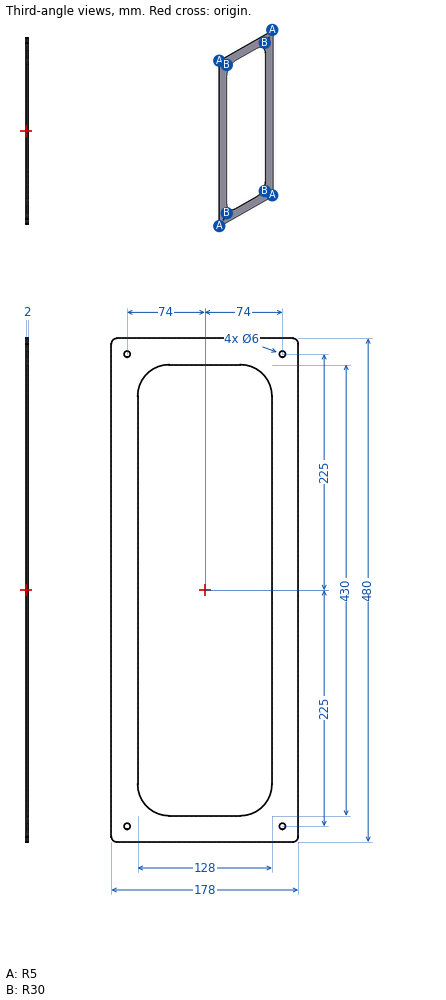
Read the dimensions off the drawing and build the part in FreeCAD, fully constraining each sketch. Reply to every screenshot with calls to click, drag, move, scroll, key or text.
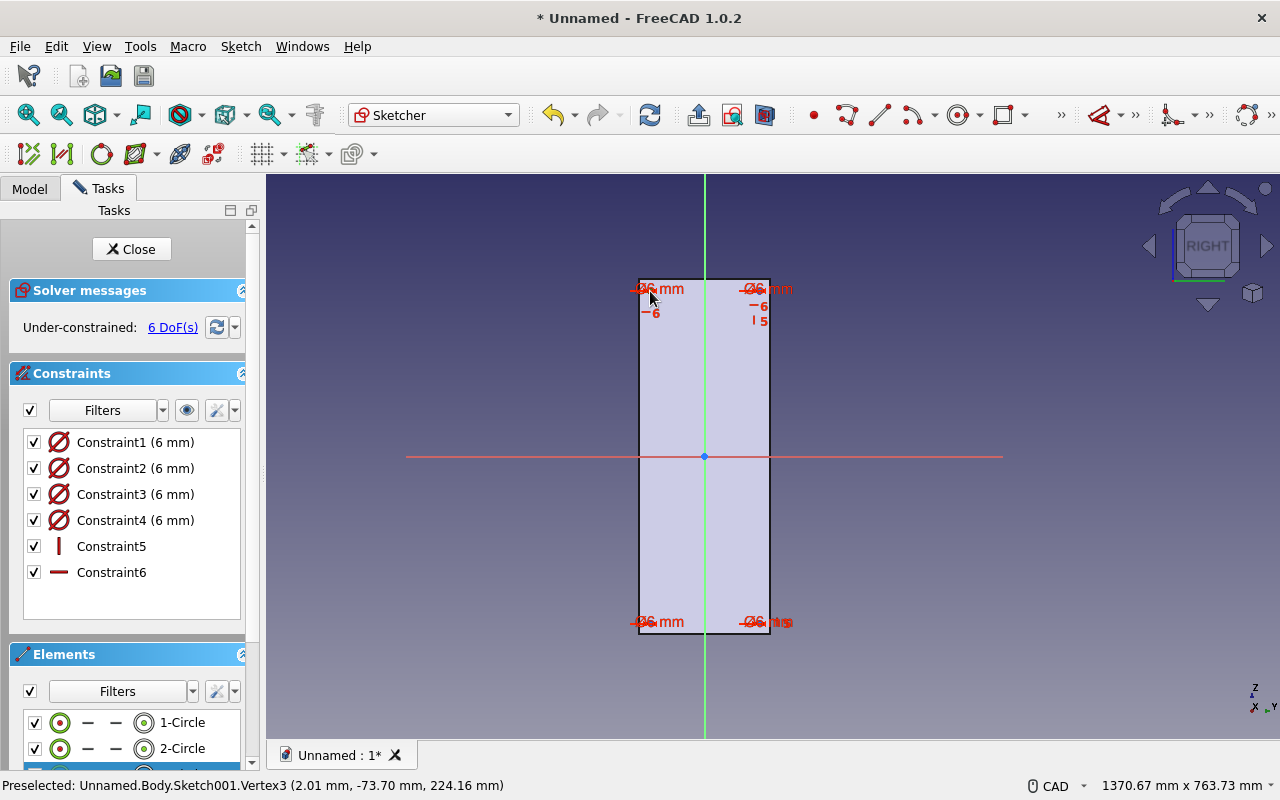
click(650, 624)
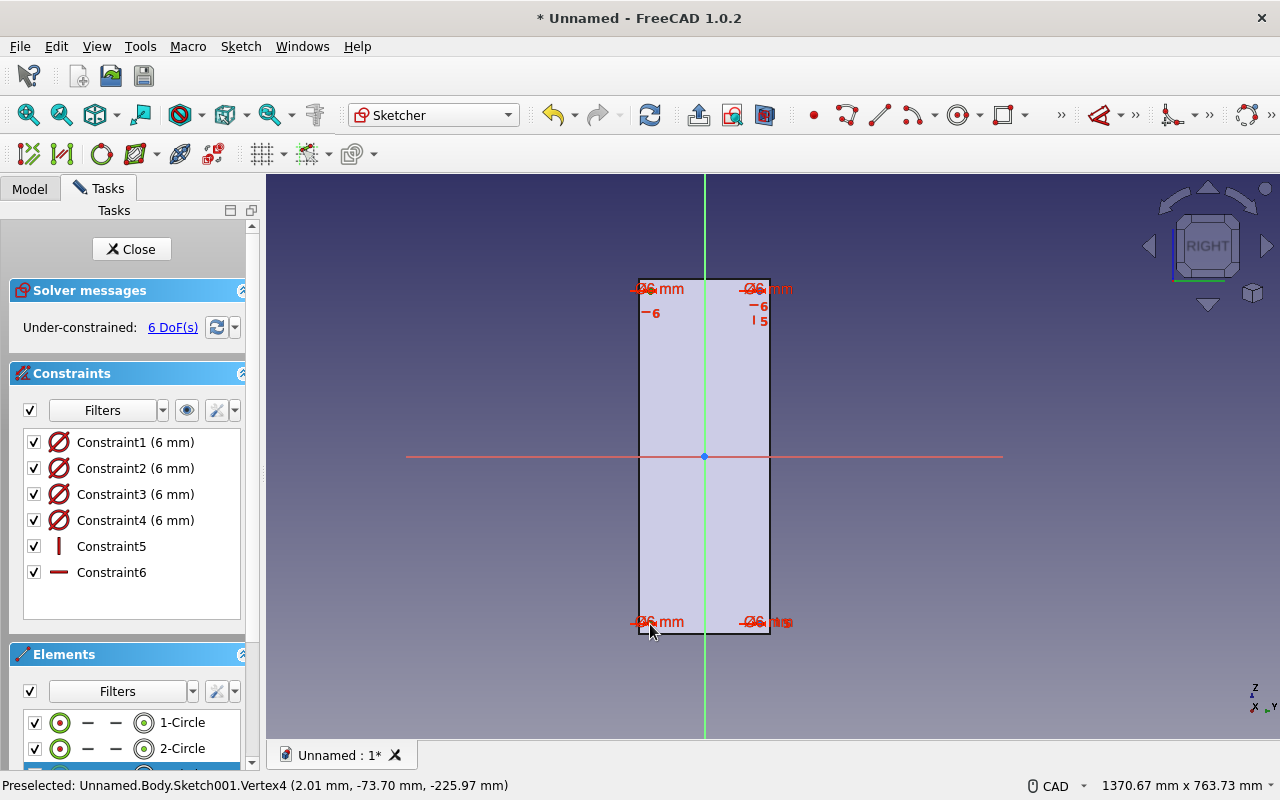
key(v)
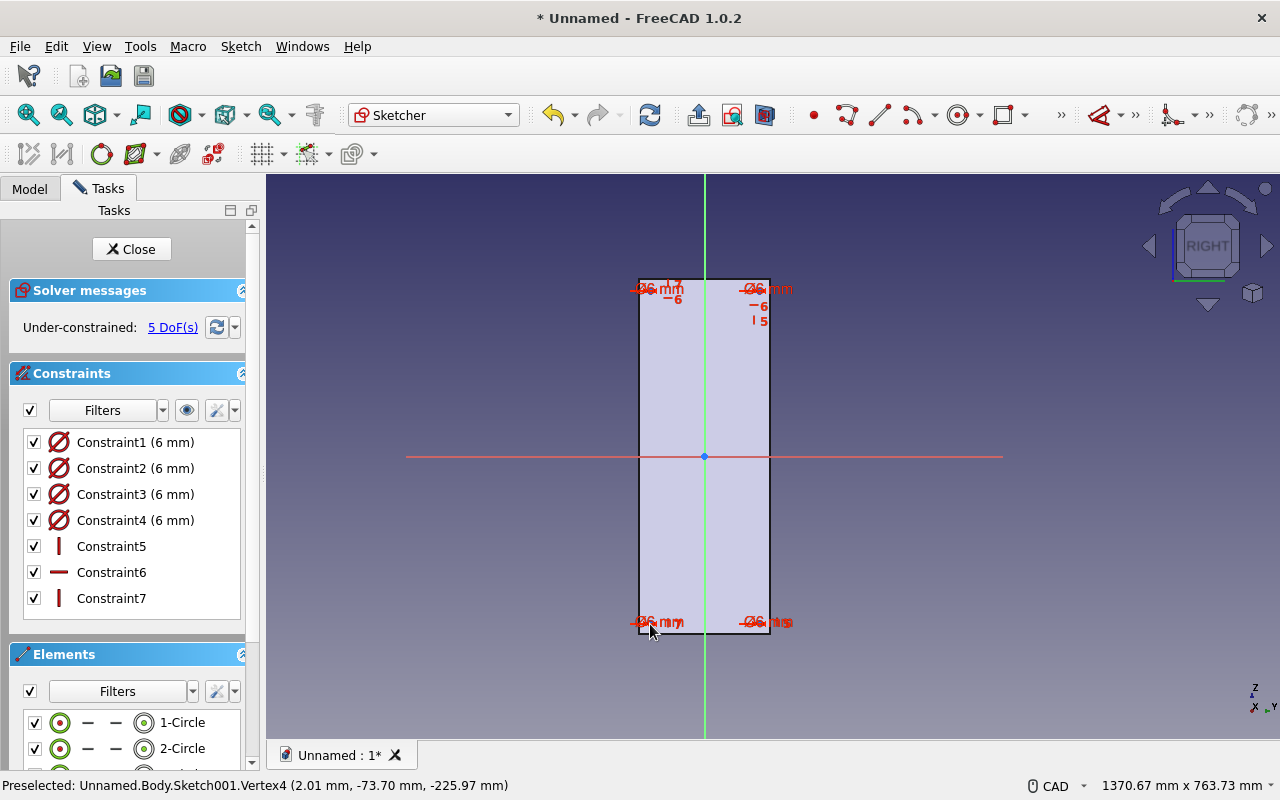
click(759, 624)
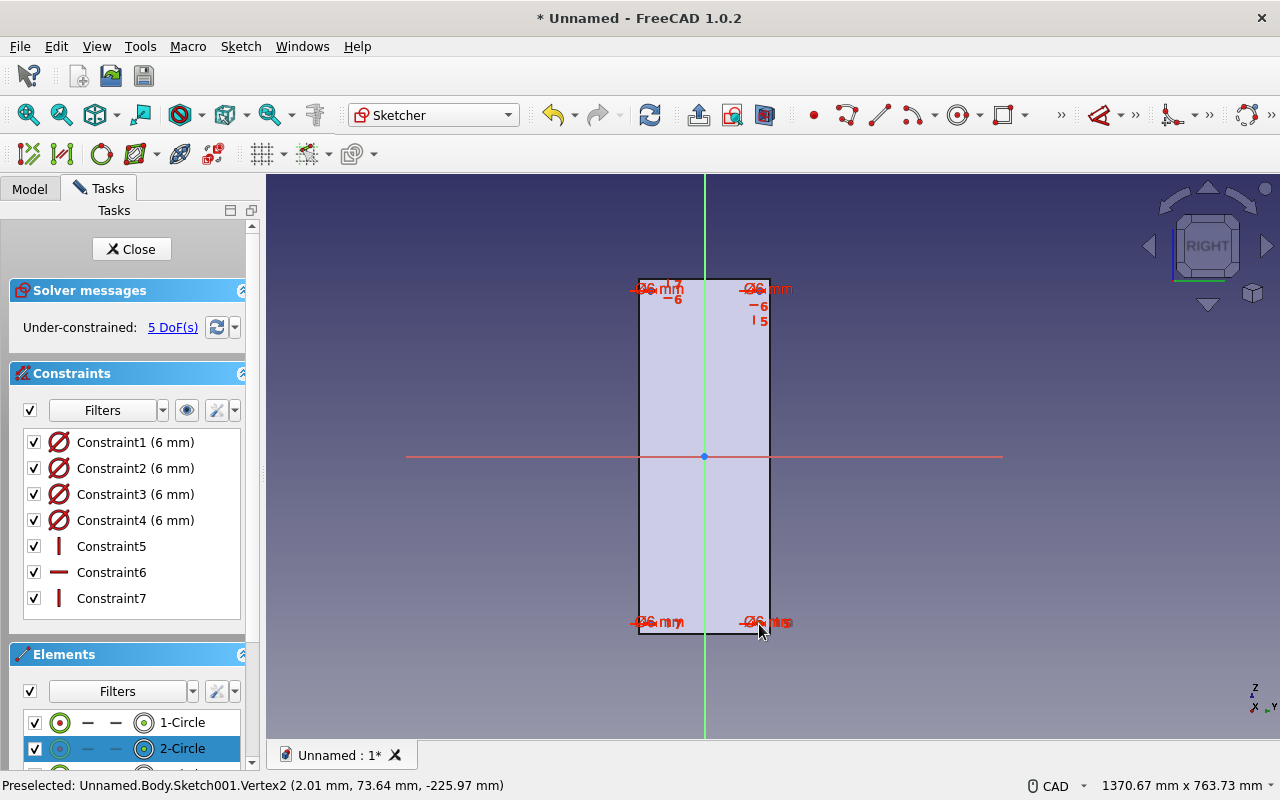
click(650, 624)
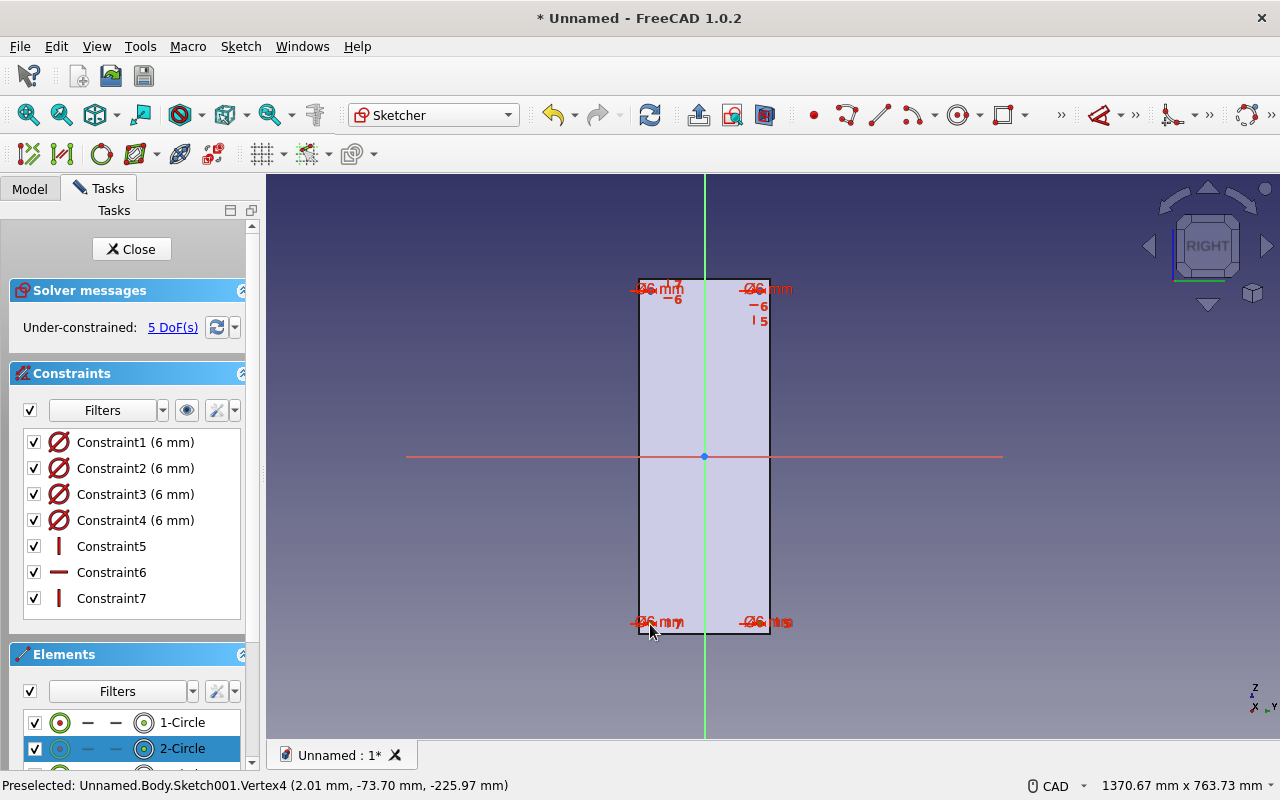
key(h)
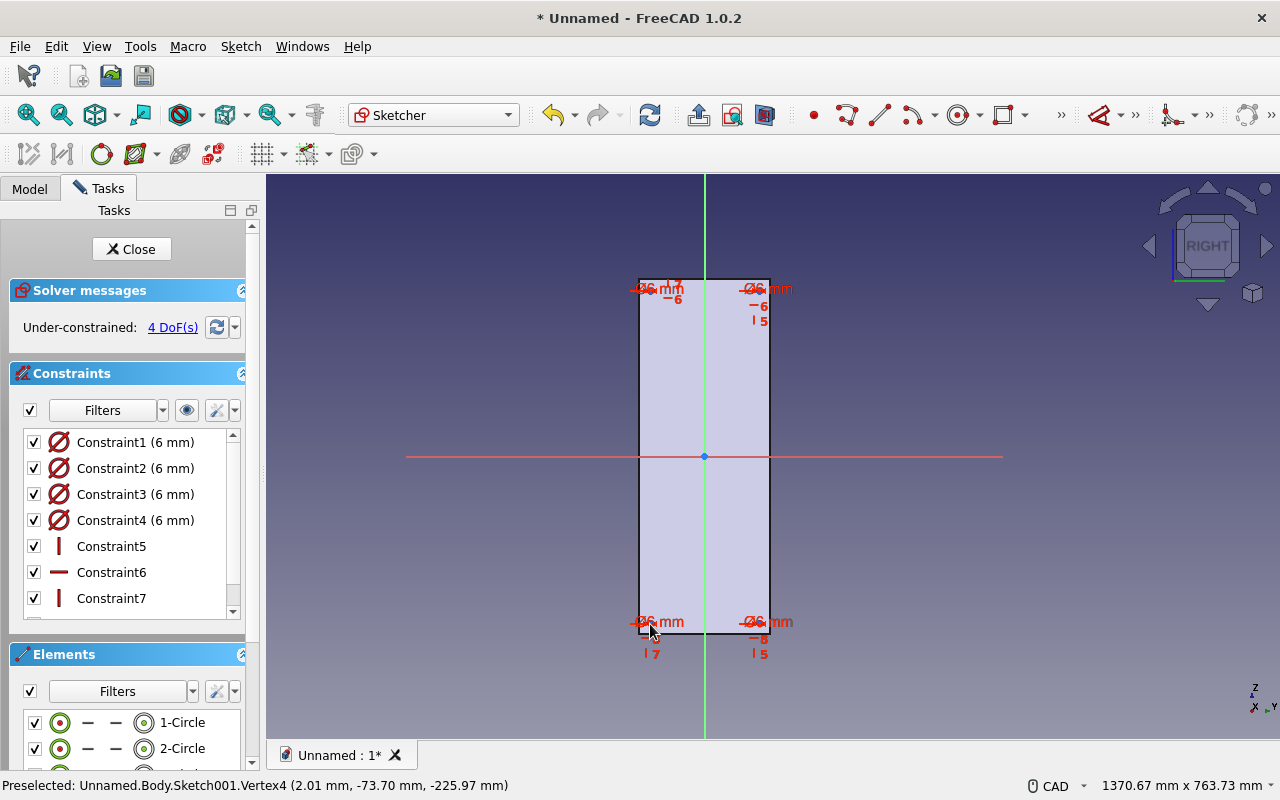
click(1098, 116)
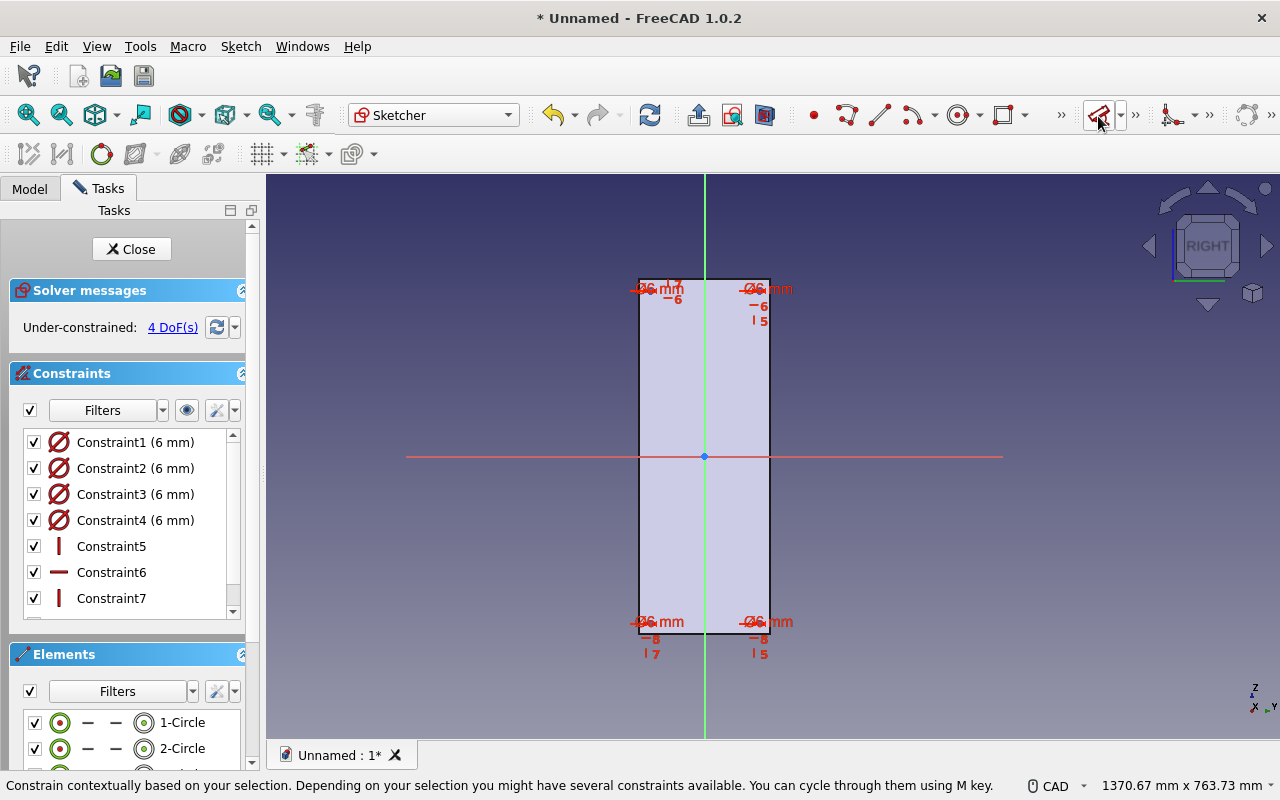
click(759, 291)
click(732, 257)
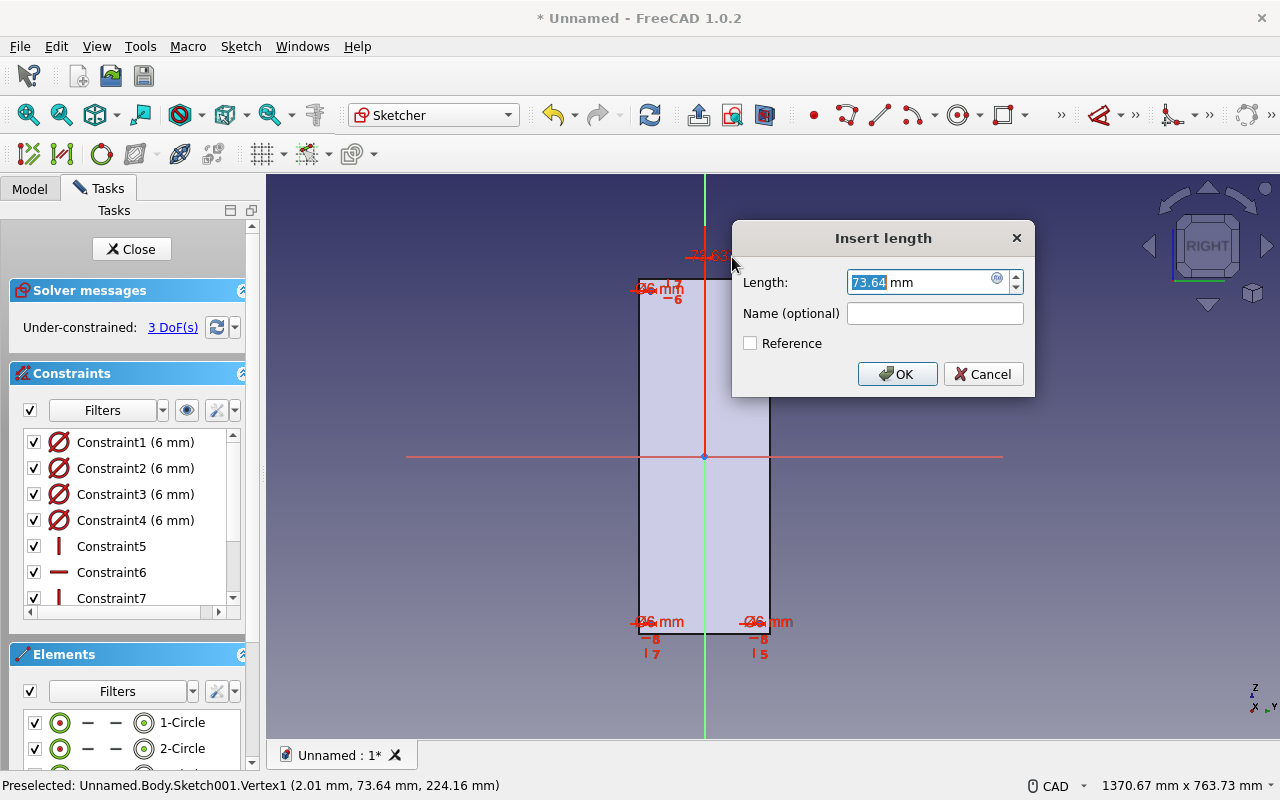
text(74)
key(Return)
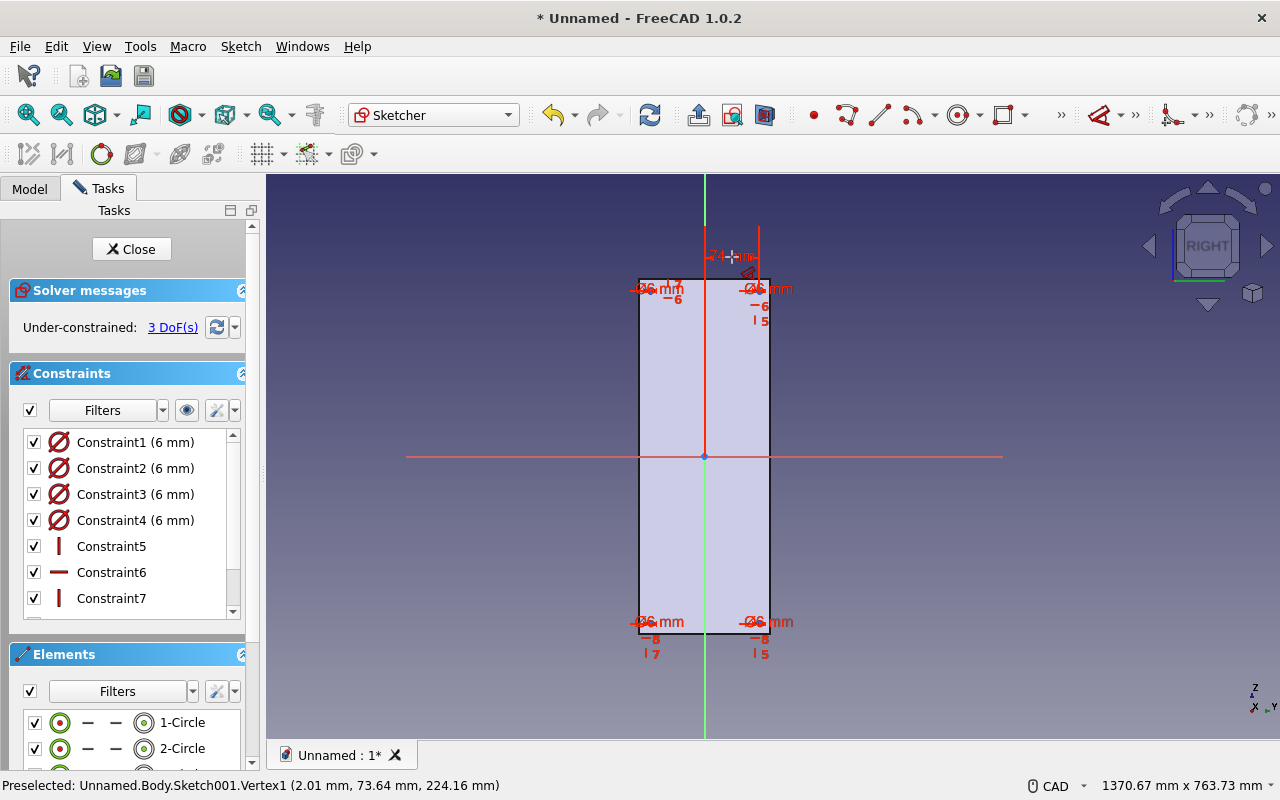
click(650, 291)
click(658, 257)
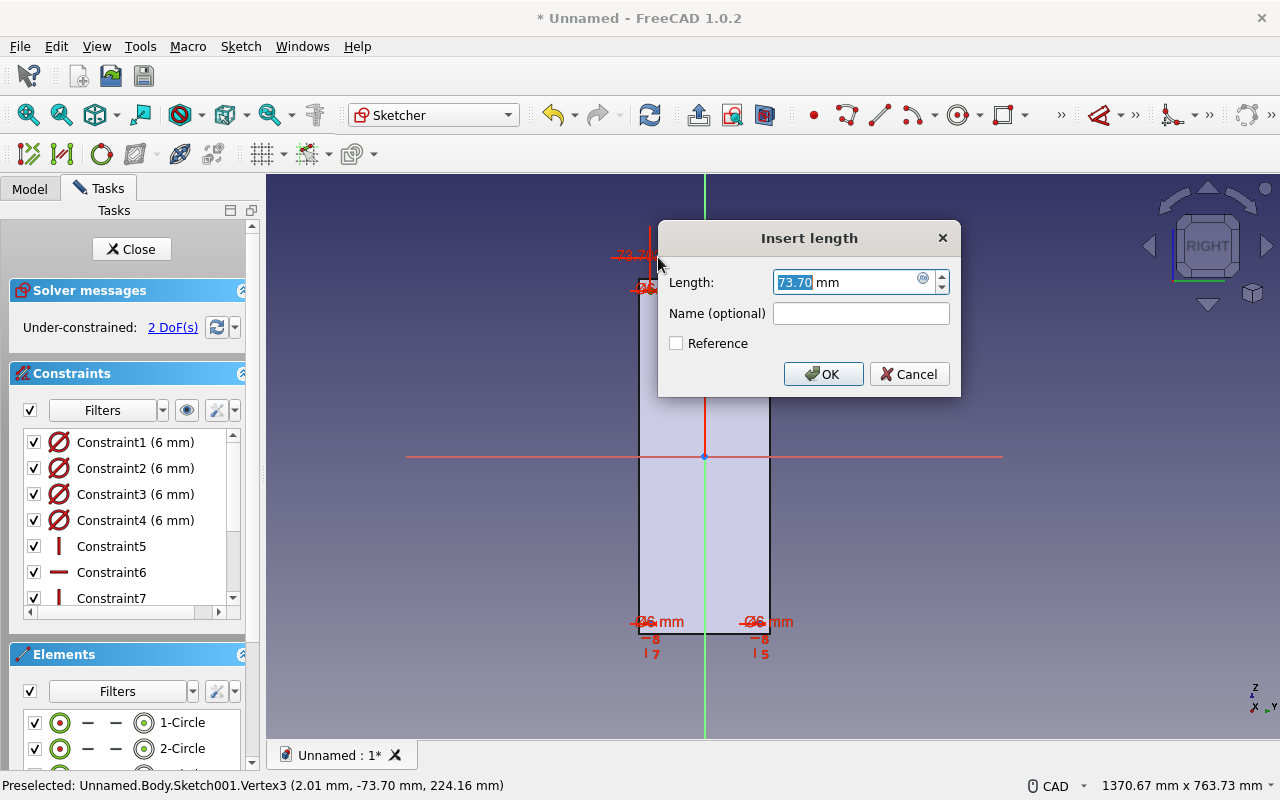
text(74)
key(Return)